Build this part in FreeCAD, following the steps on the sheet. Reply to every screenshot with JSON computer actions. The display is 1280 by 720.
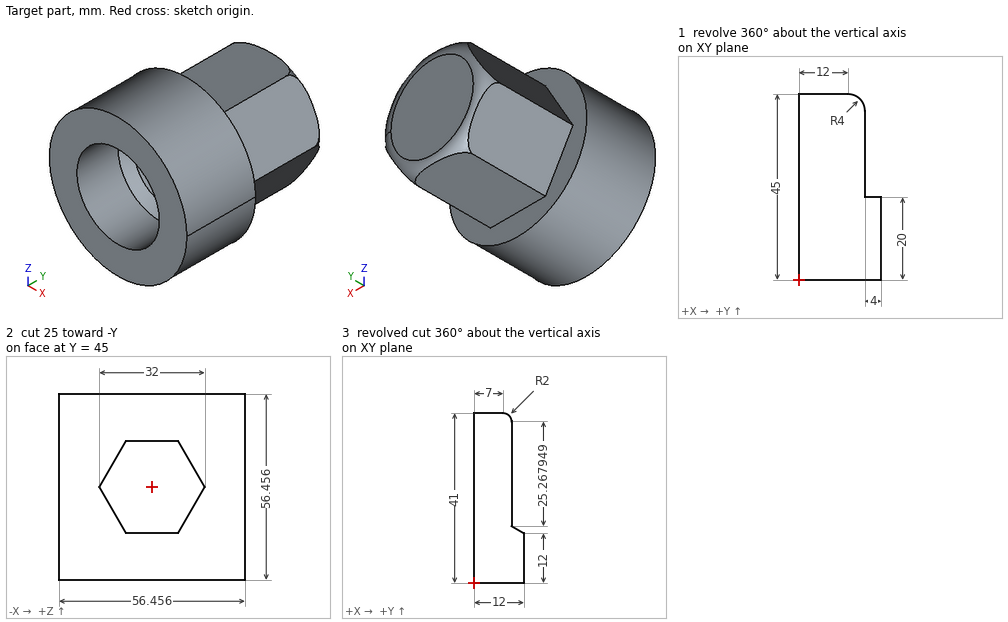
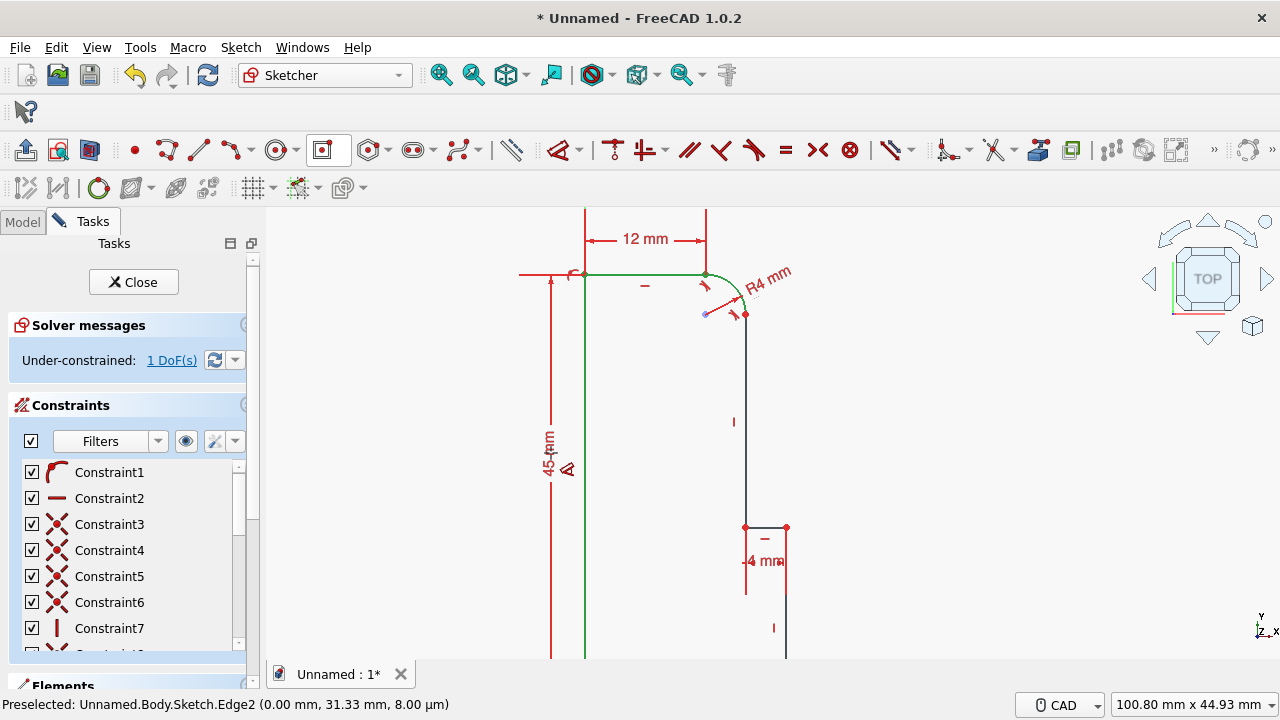
{"action": "left_click", "coordinate": [786, 587]}
{"action": "left_click", "coordinate": [820, 603]}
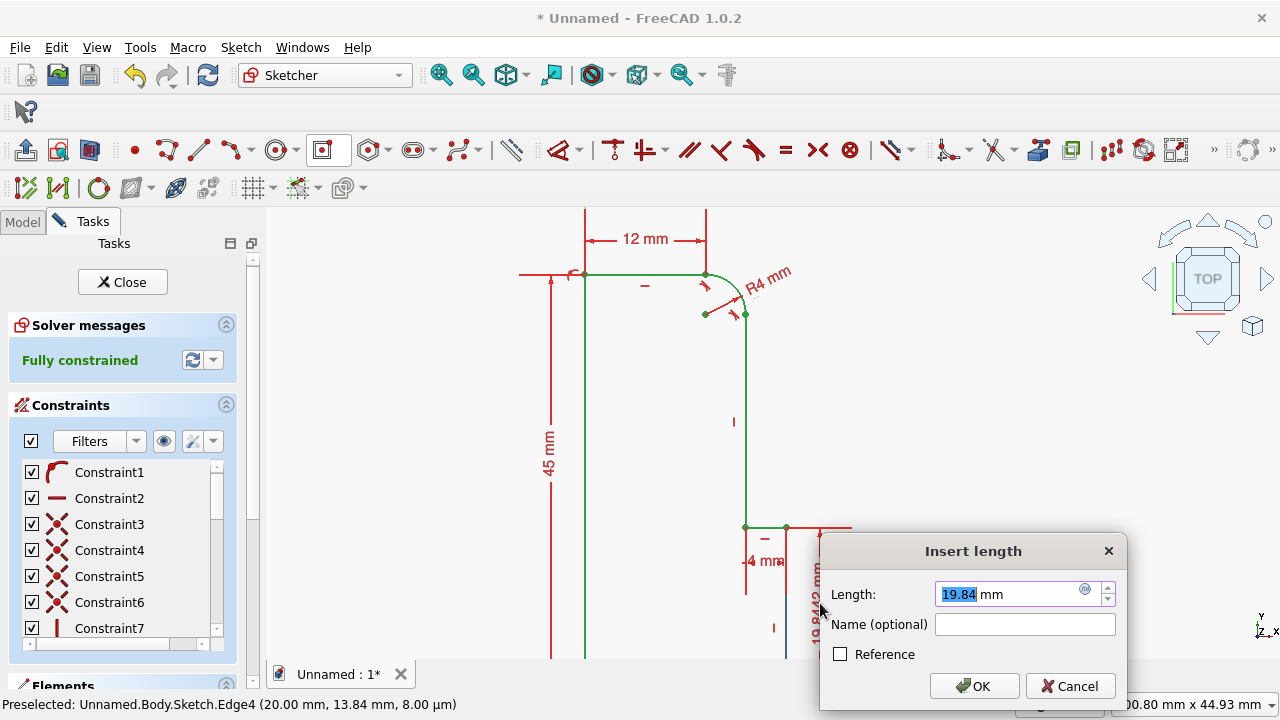
{"action": "type", "text": "20"}
{"action": "key", "text": "Return"}
{"action": "key", "text": "Escape"}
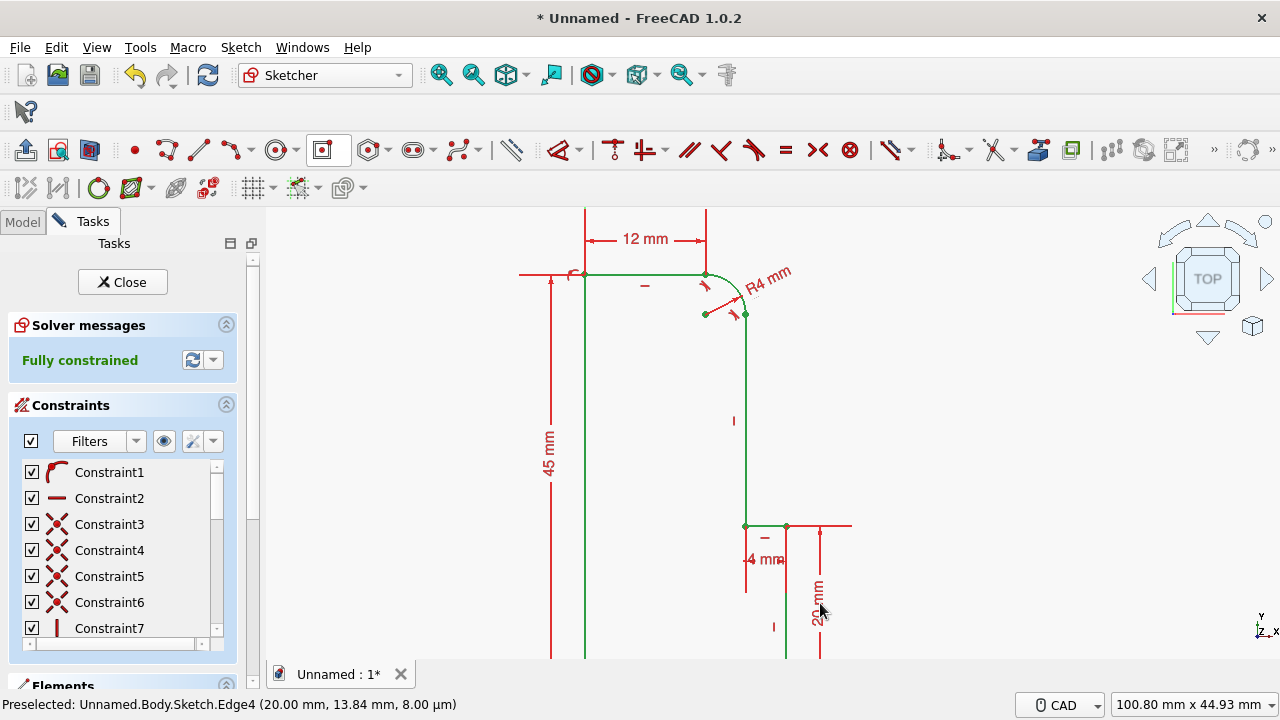
{"action": "left_click", "coordinate": [123, 282]}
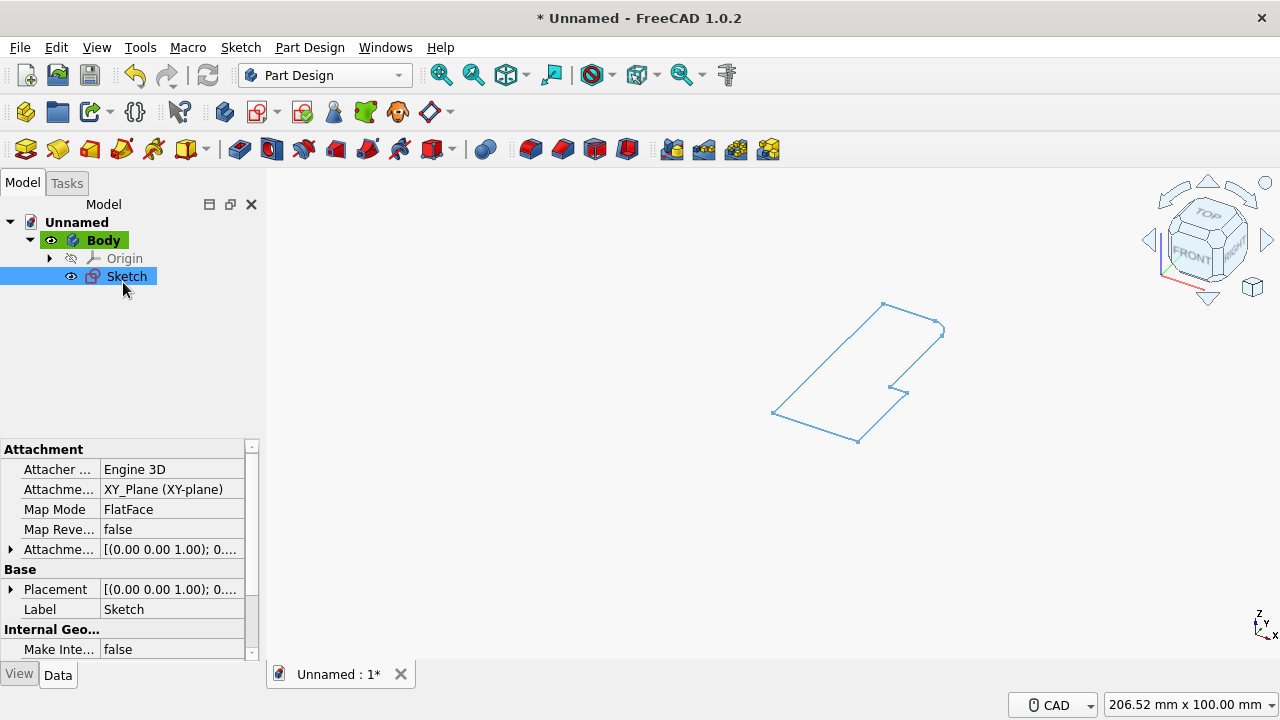
{"action": "left_click", "coordinate": [58, 150]}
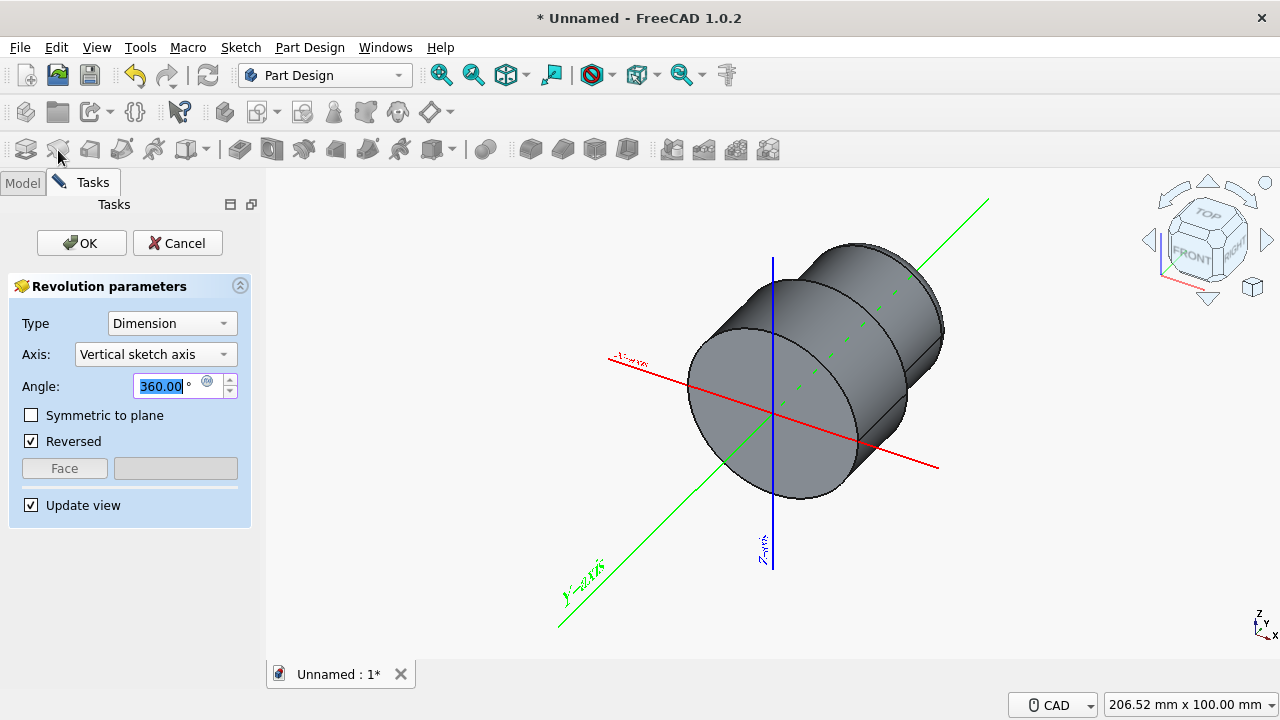
{"action": "left_click", "coordinate": [82, 243]}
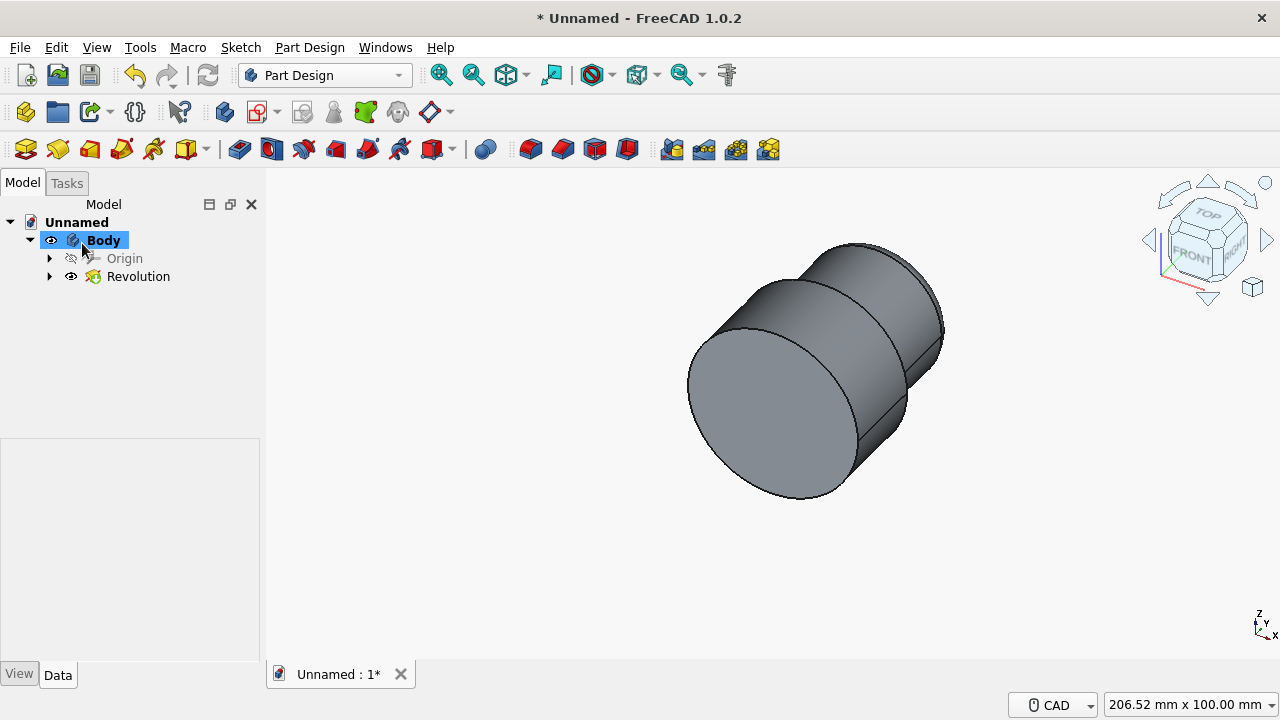
{"action": "key", "text": "4"}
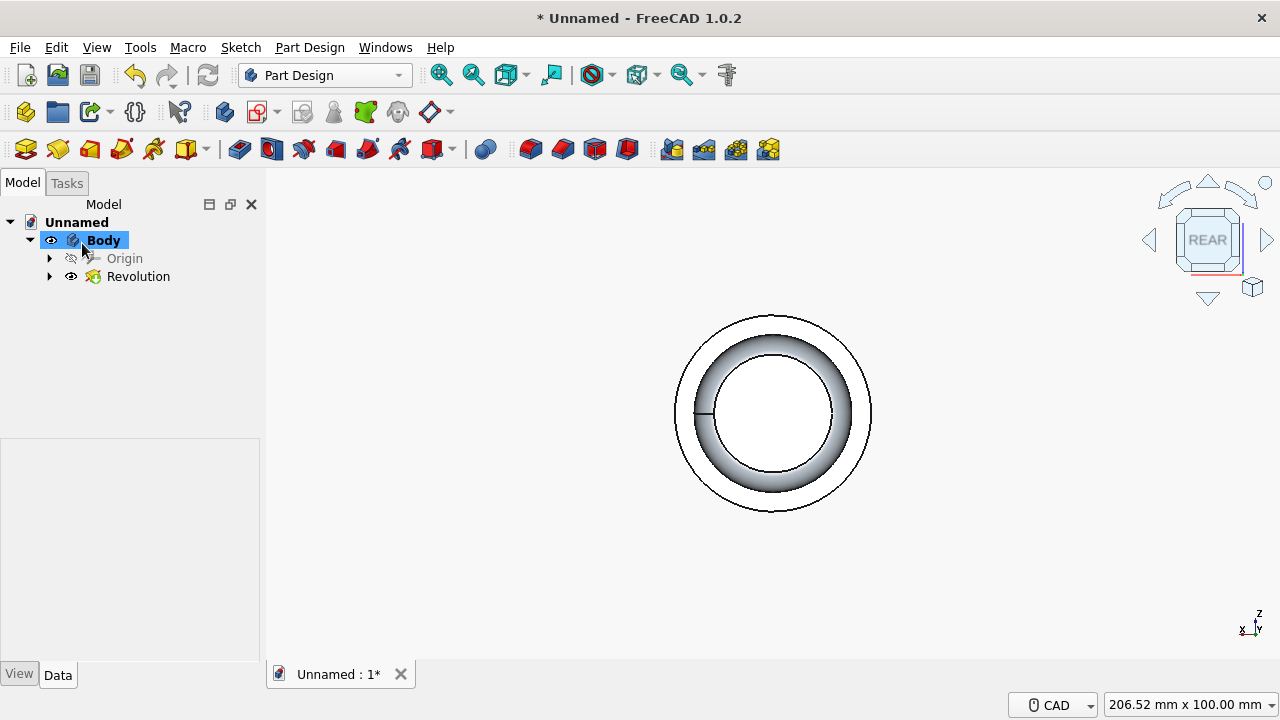
{"action": "left_click", "coordinate": [442, 76]}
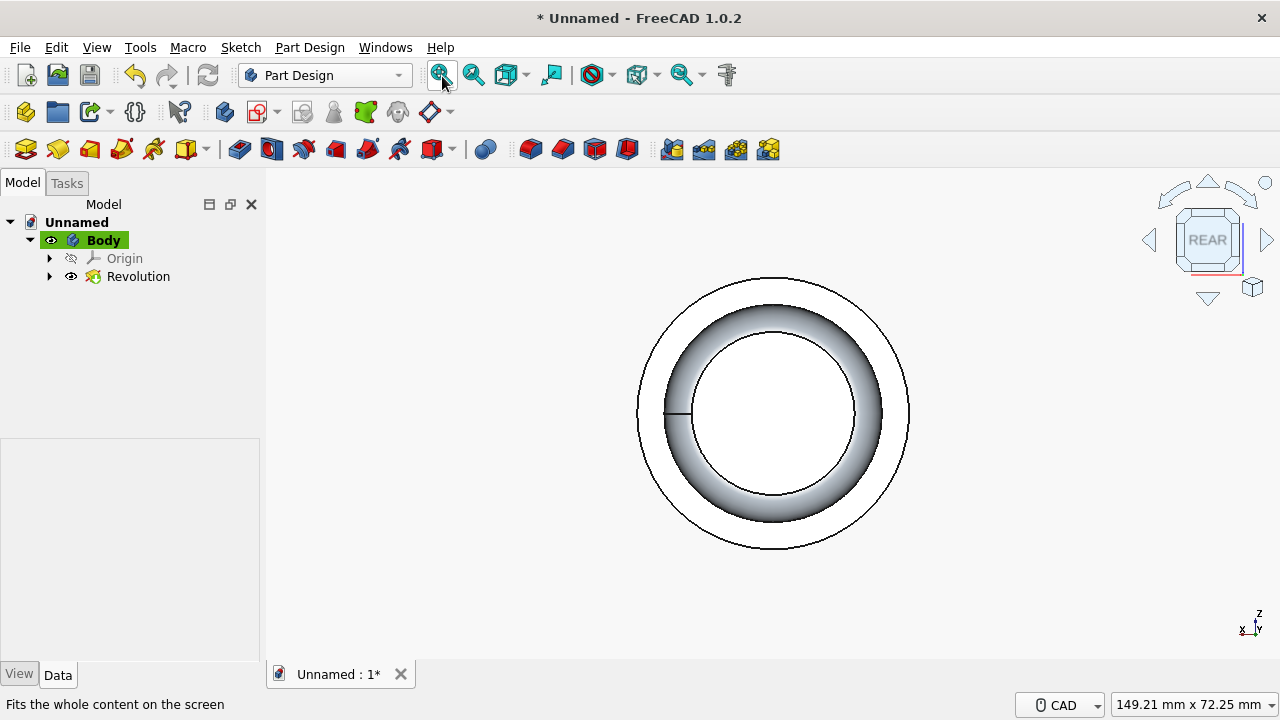
{"action": "left_click", "coordinate": [773, 413]}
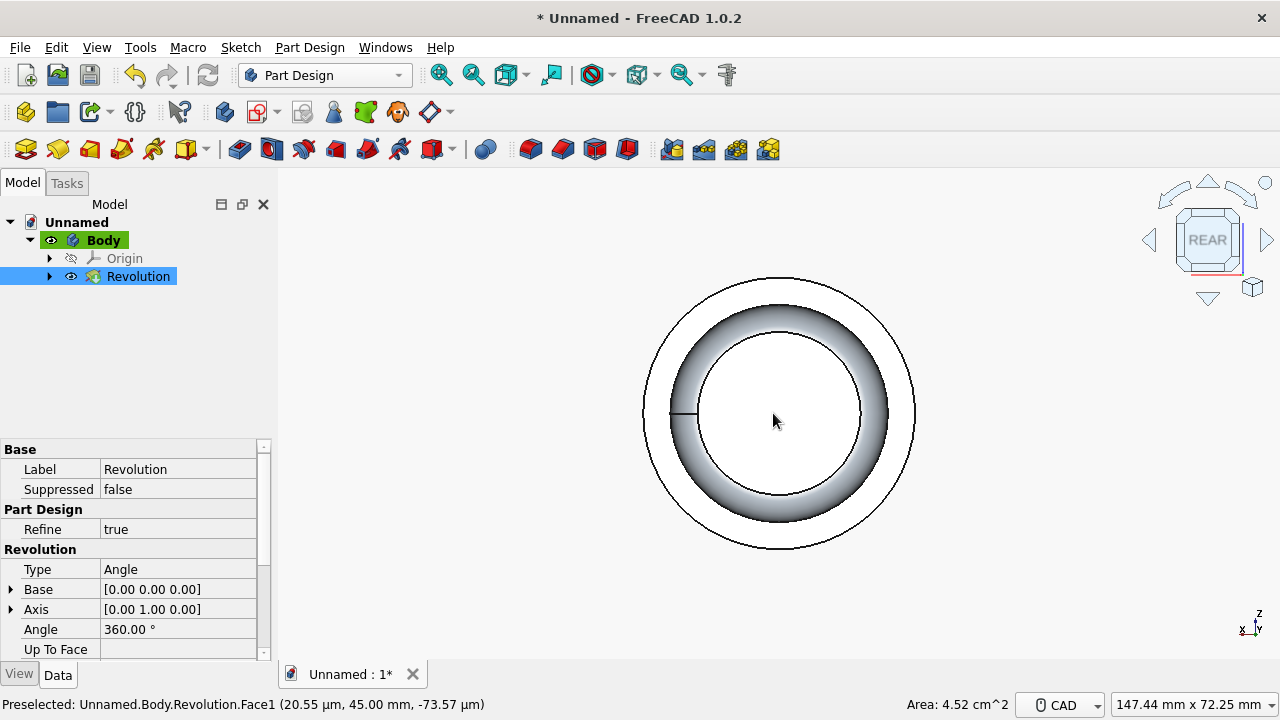
{"action": "left_click", "coordinate": [258, 112]}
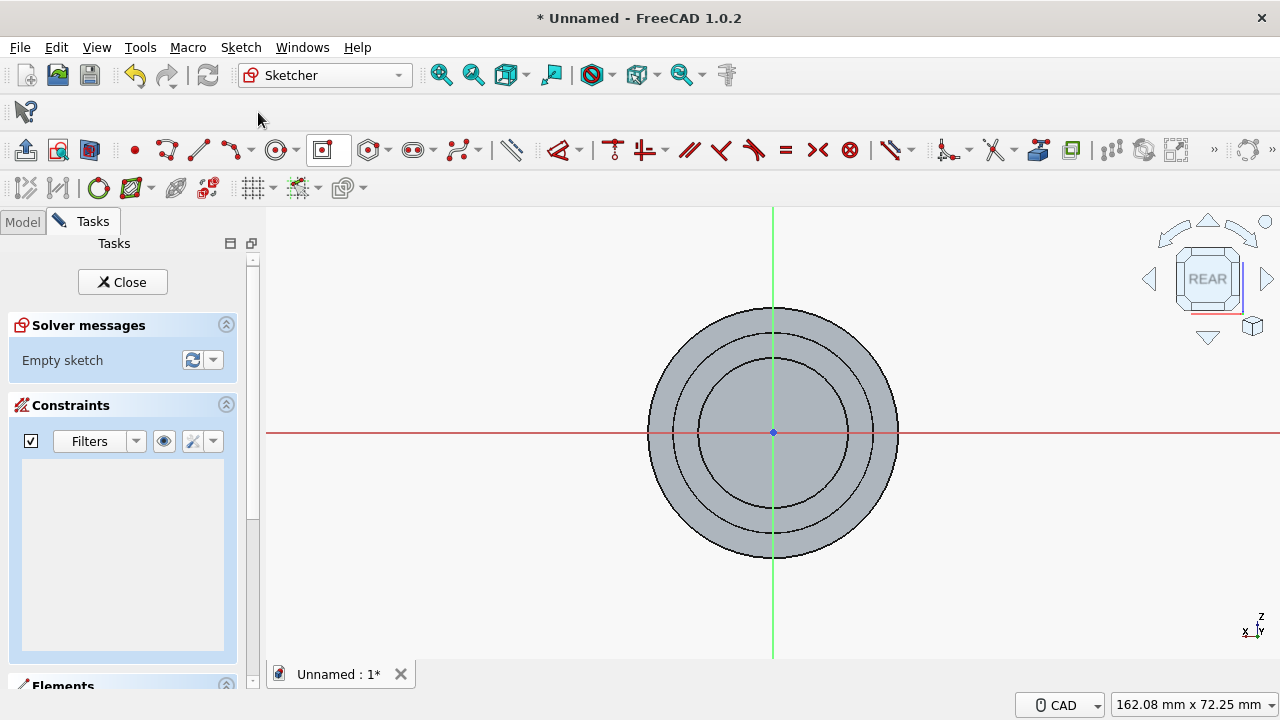
{"action": "scroll", "coordinate": [395, 433], "scroll_direction": "down", "scroll_amount": 1}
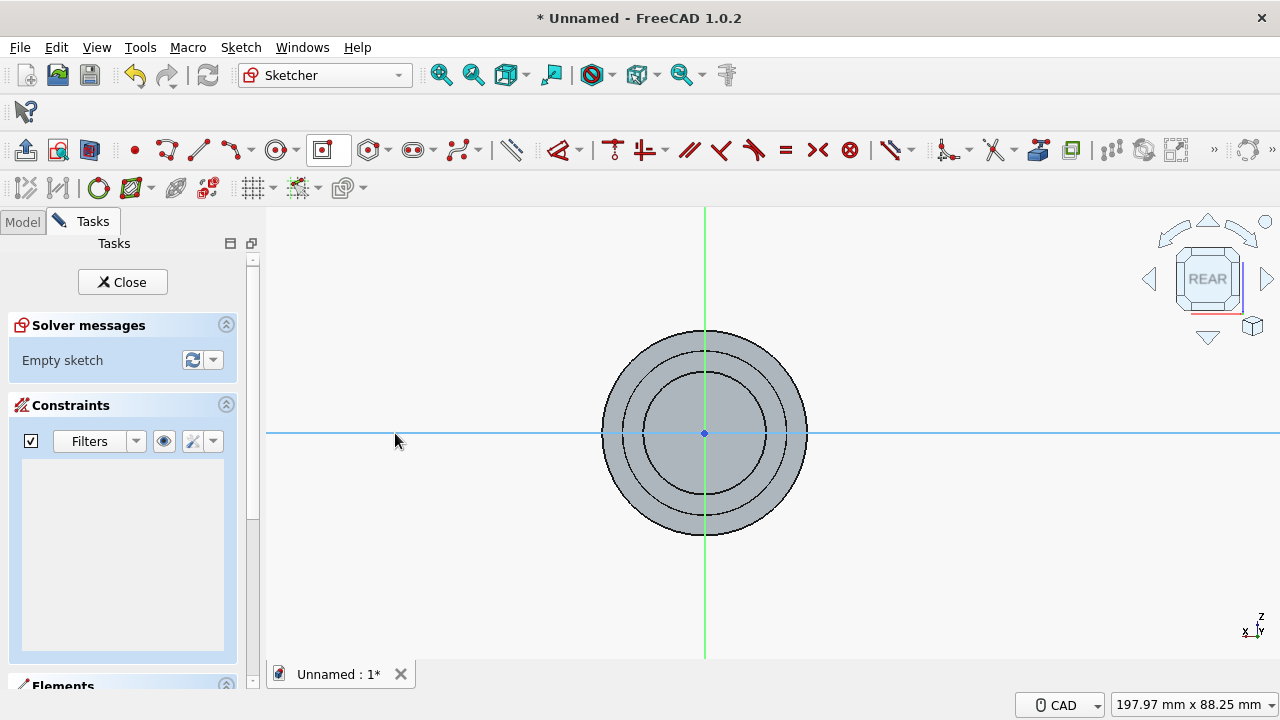
{"action": "key", "text": "g v"}